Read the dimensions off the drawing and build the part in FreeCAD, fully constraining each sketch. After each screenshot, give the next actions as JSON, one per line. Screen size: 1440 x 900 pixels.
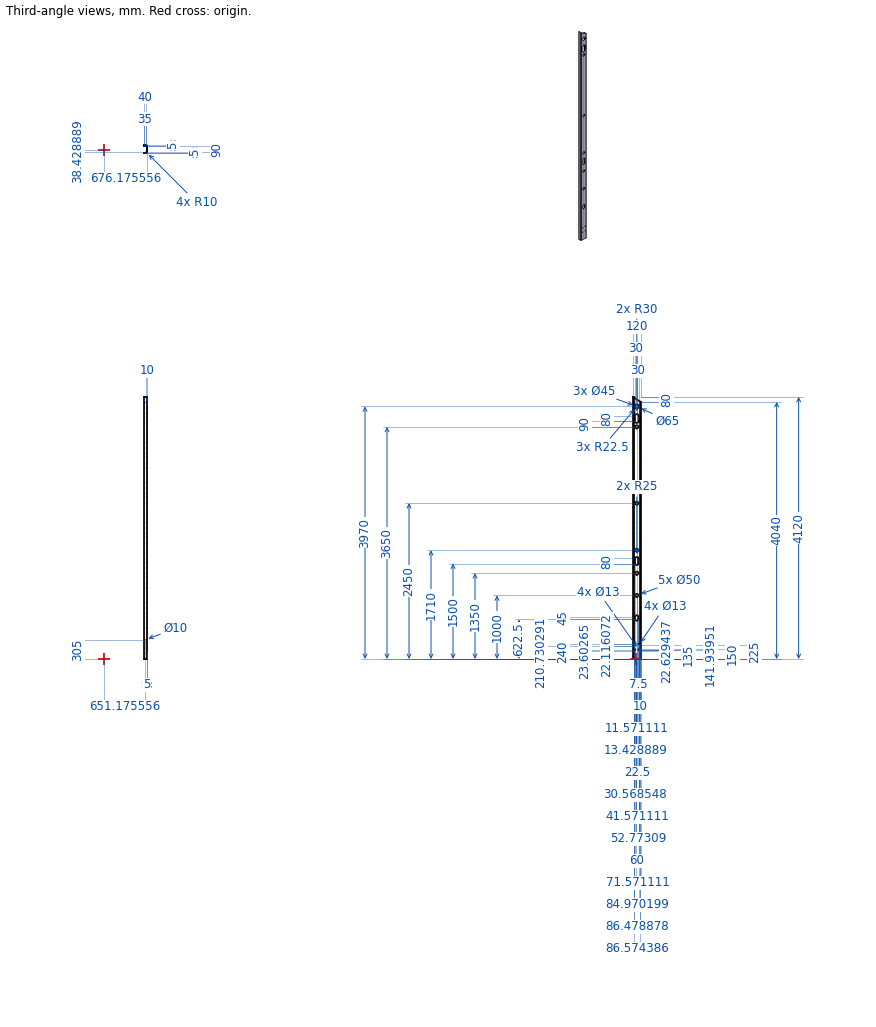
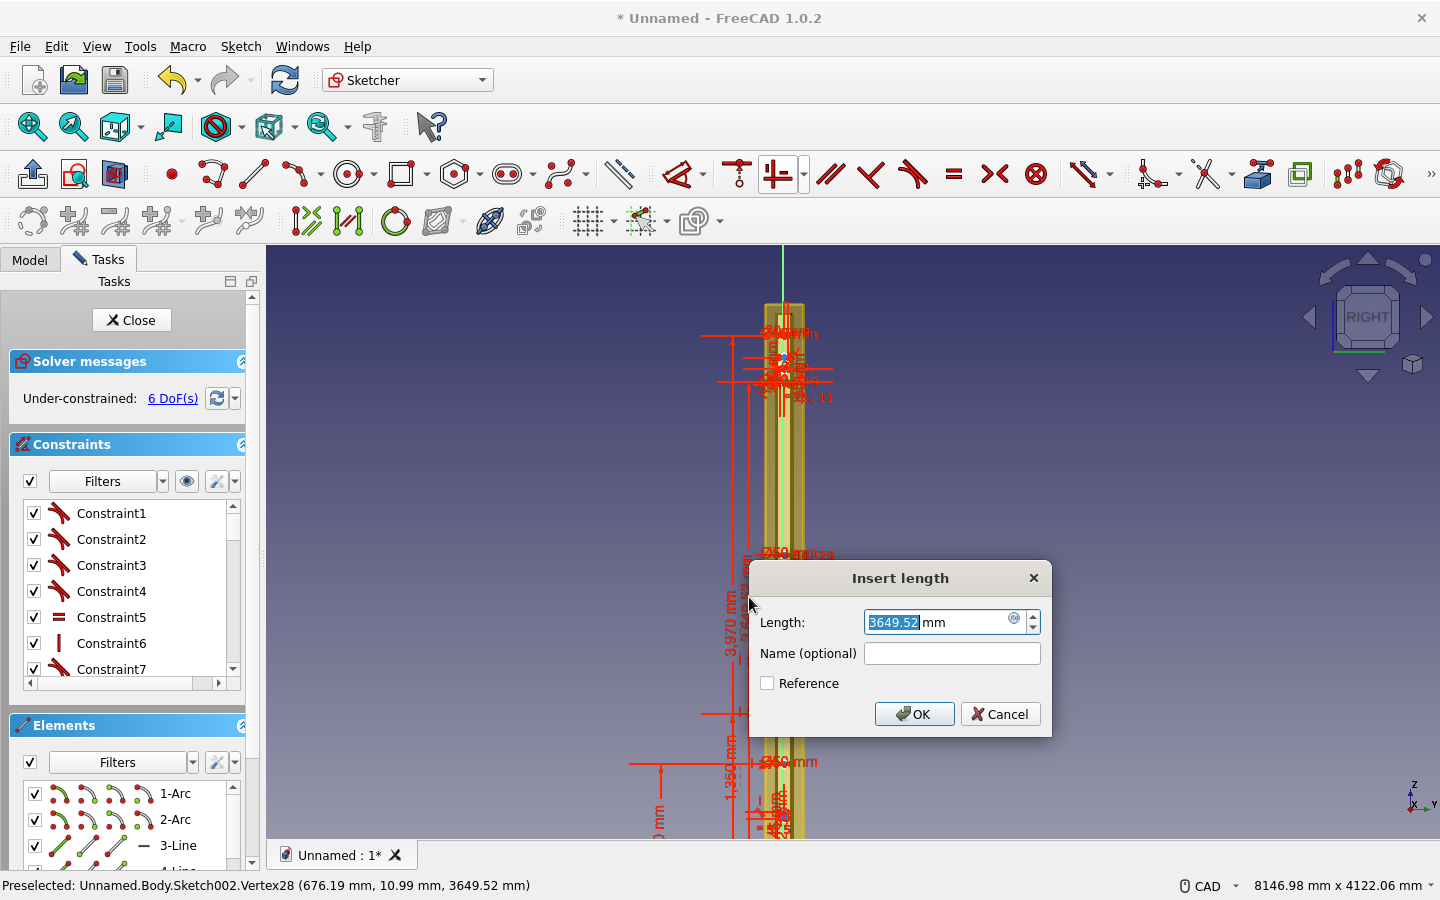
{"action": "type", "text": "3650"}
{"action": "key", "text": "Return"}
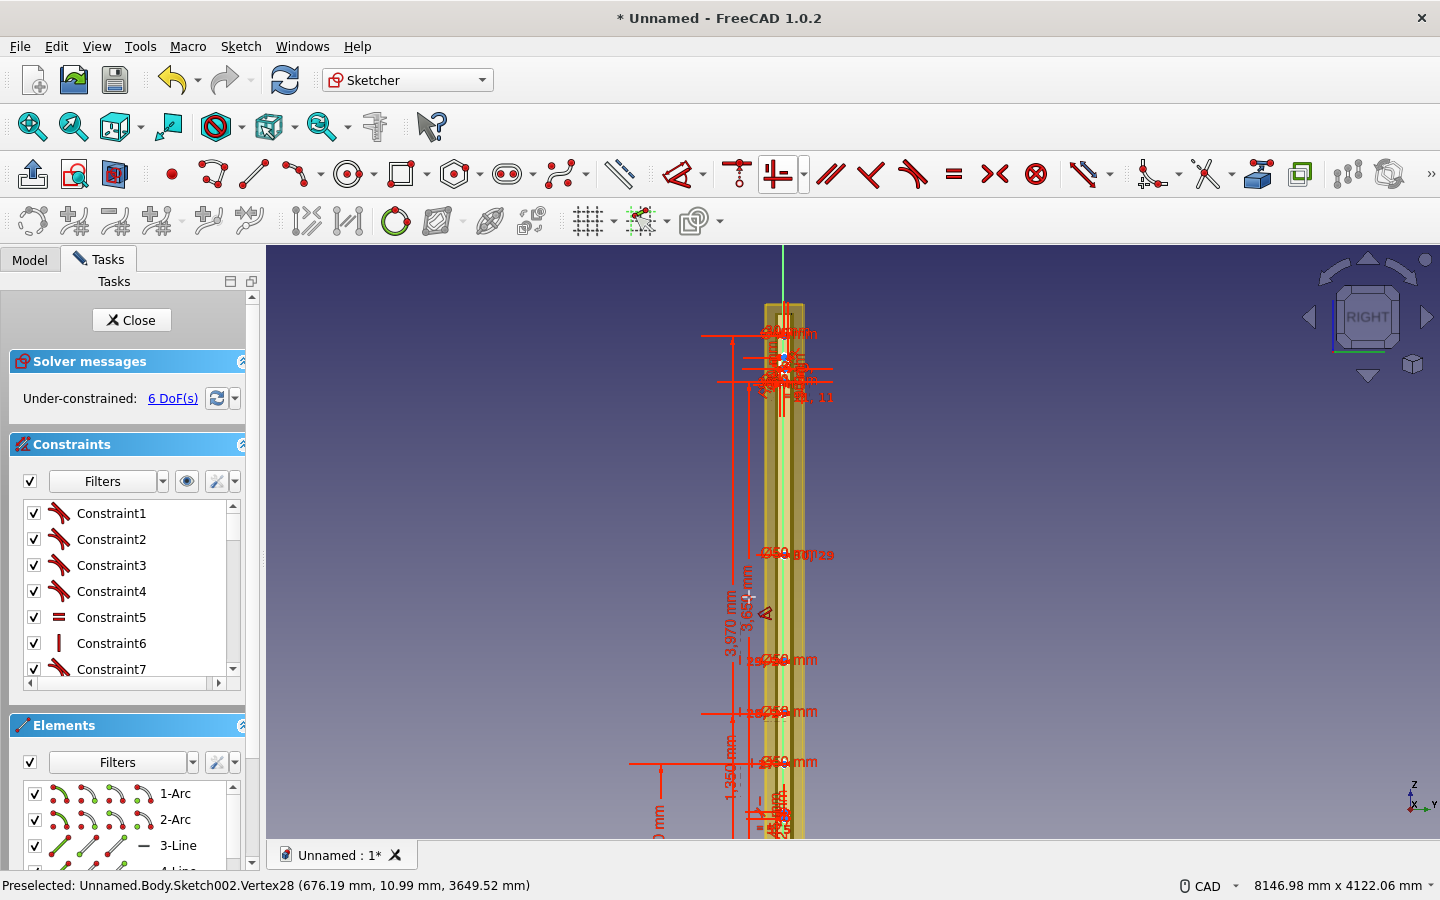
{"action": "left_click", "coordinate": [784, 662]}
{"action": "left_click", "coordinate": [749, 736]}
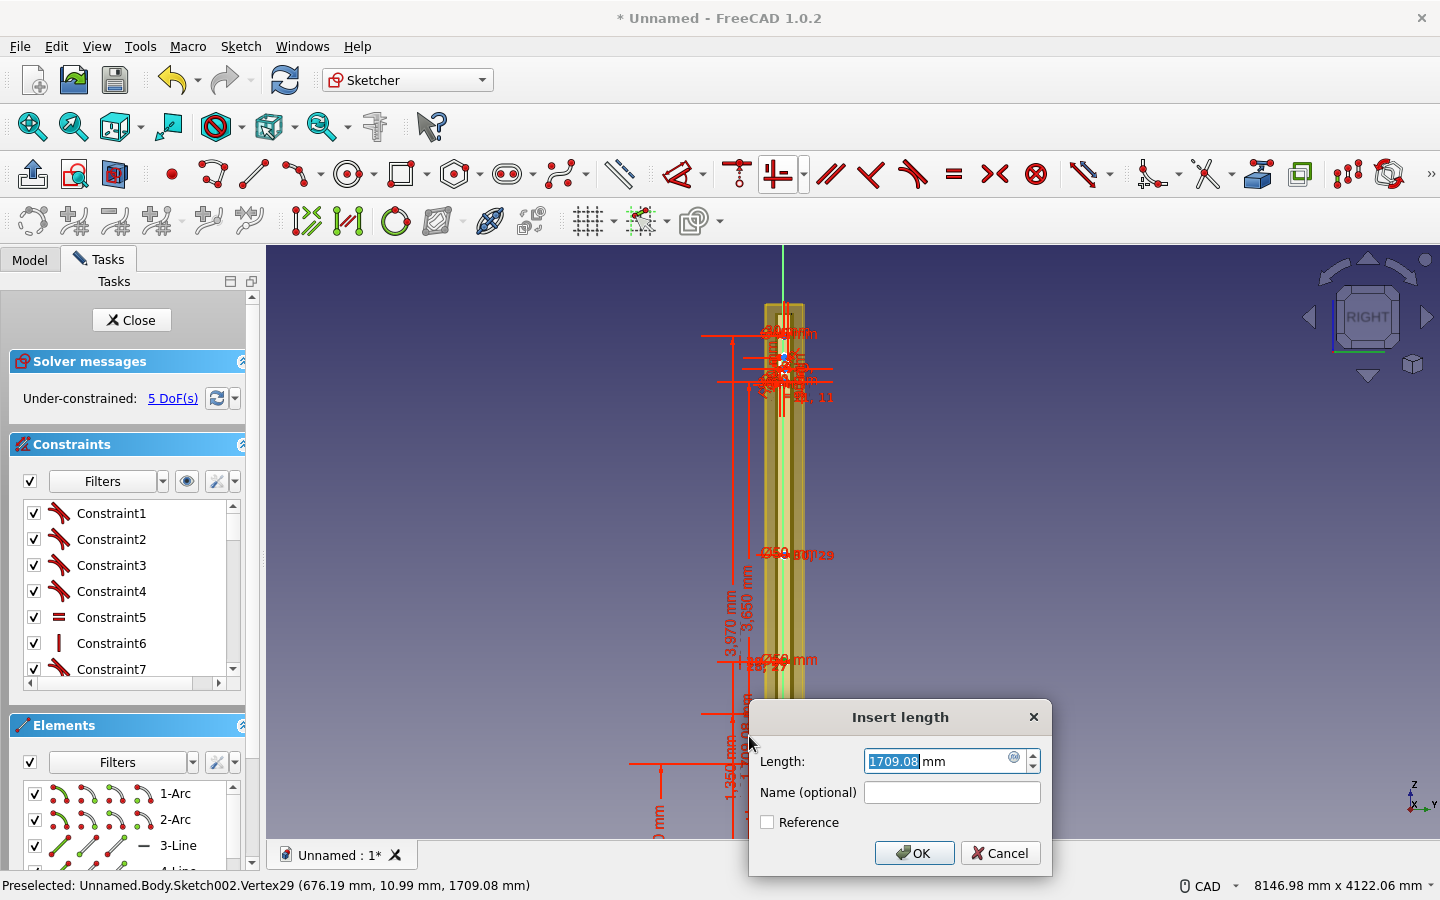
{"action": "type", "text": "1710"}
{"action": "key", "text": "Return"}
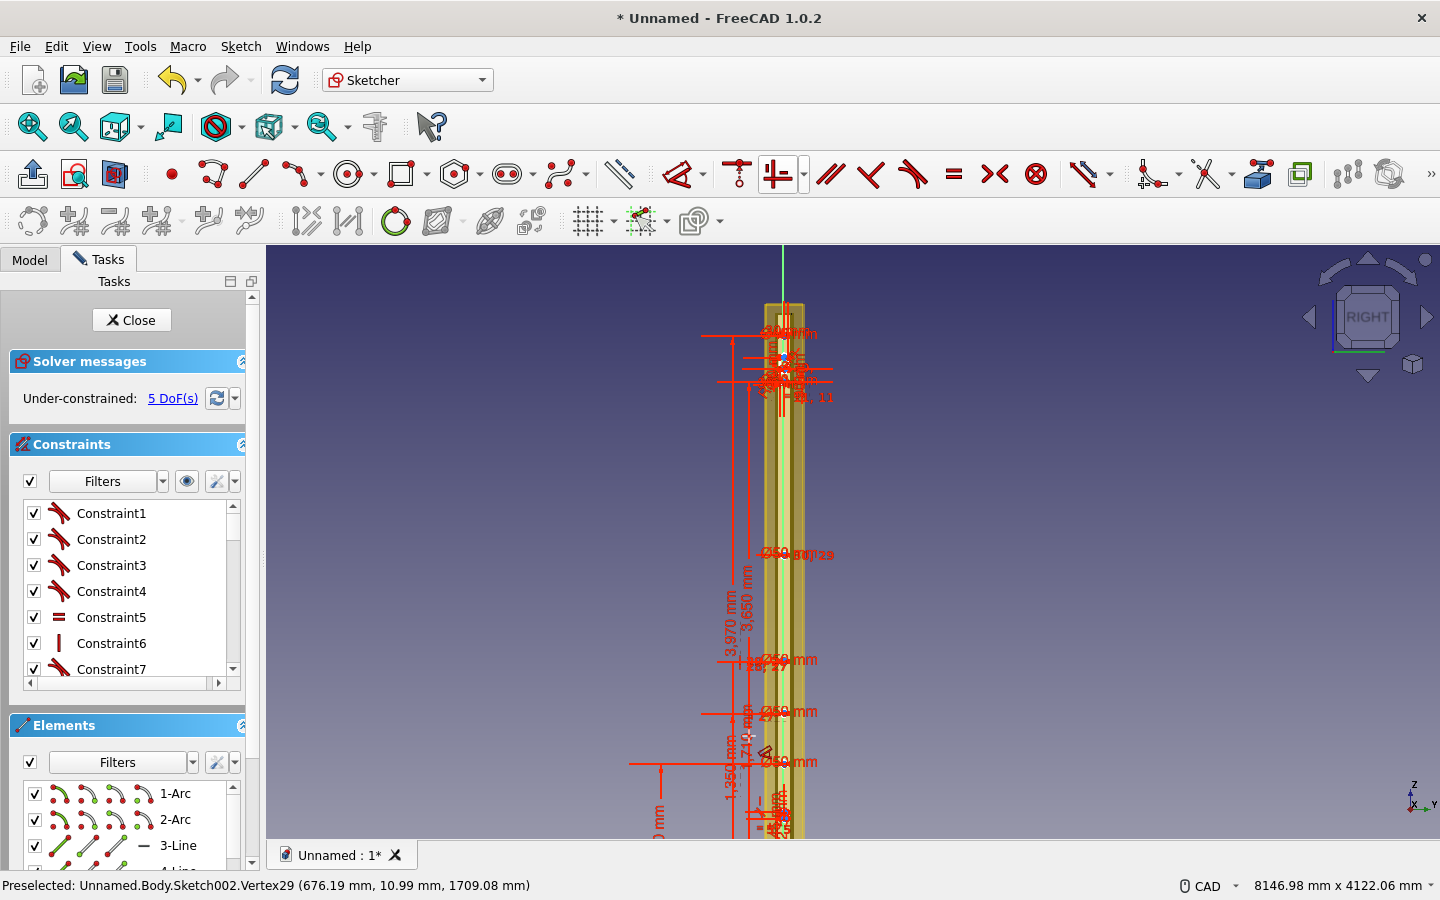
{"action": "left_click", "coordinate": [784, 555]}
{"action": "left_click", "coordinate": [749, 683]}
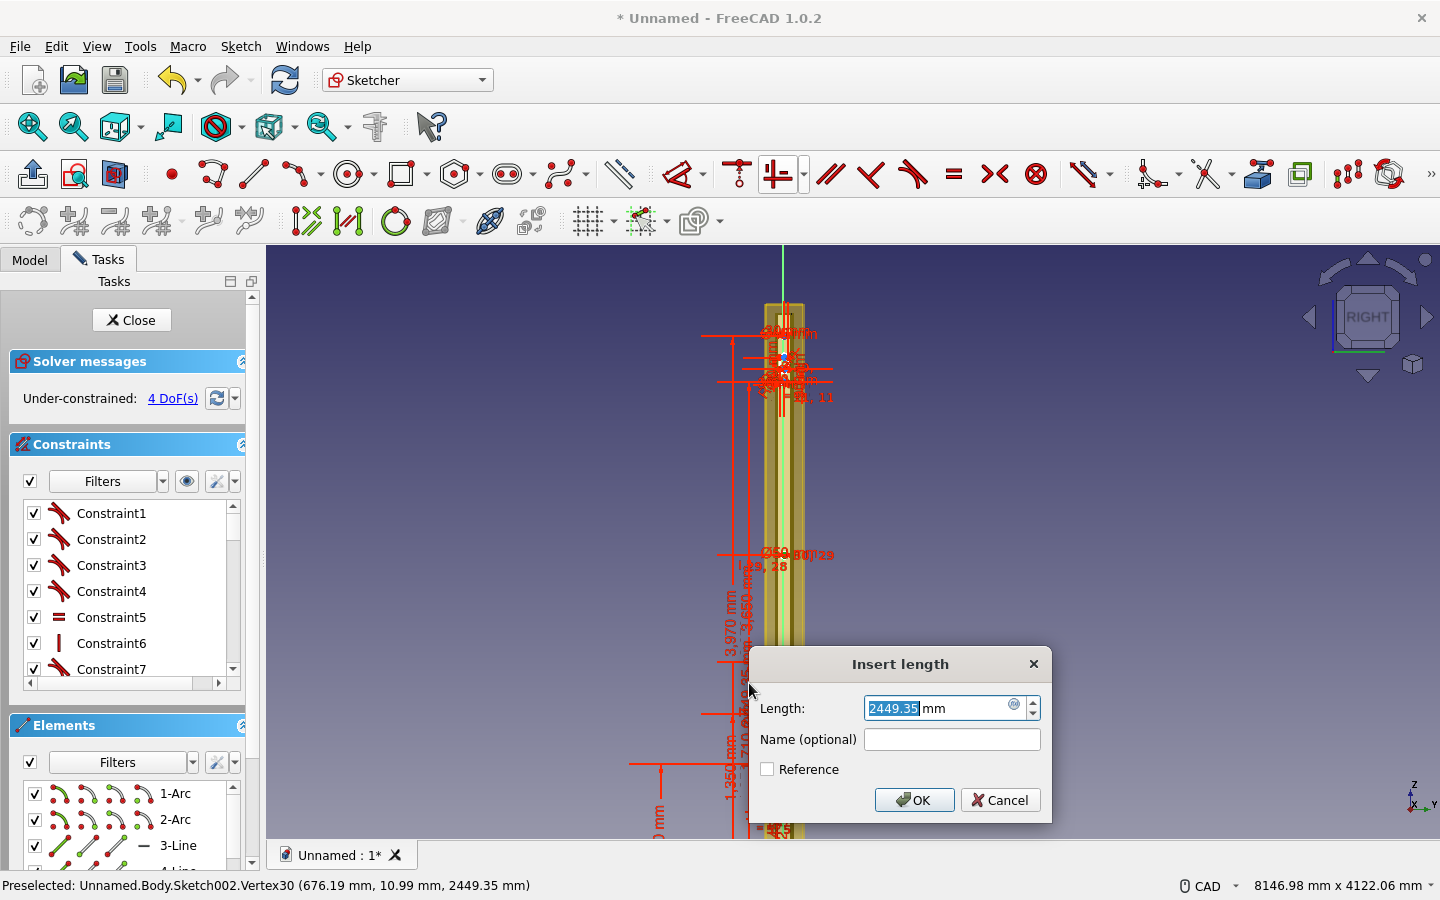
{"action": "type", "text": "2450"}
{"action": "key", "text": "Return"}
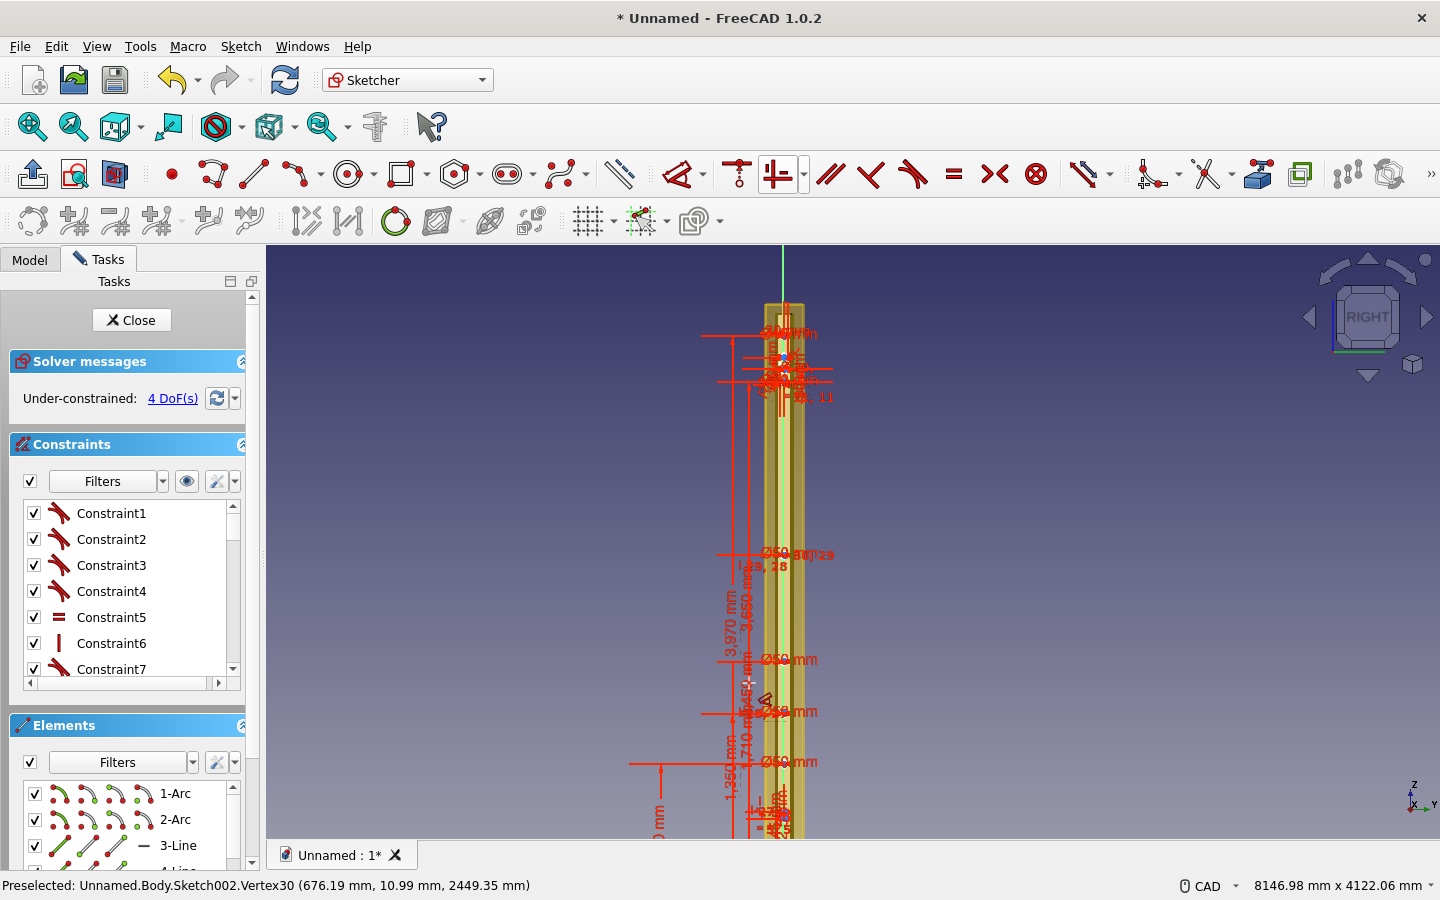
{"action": "scroll", "coordinate": [785, 382], "scroll_direction": "down", "scroll_amount": 2}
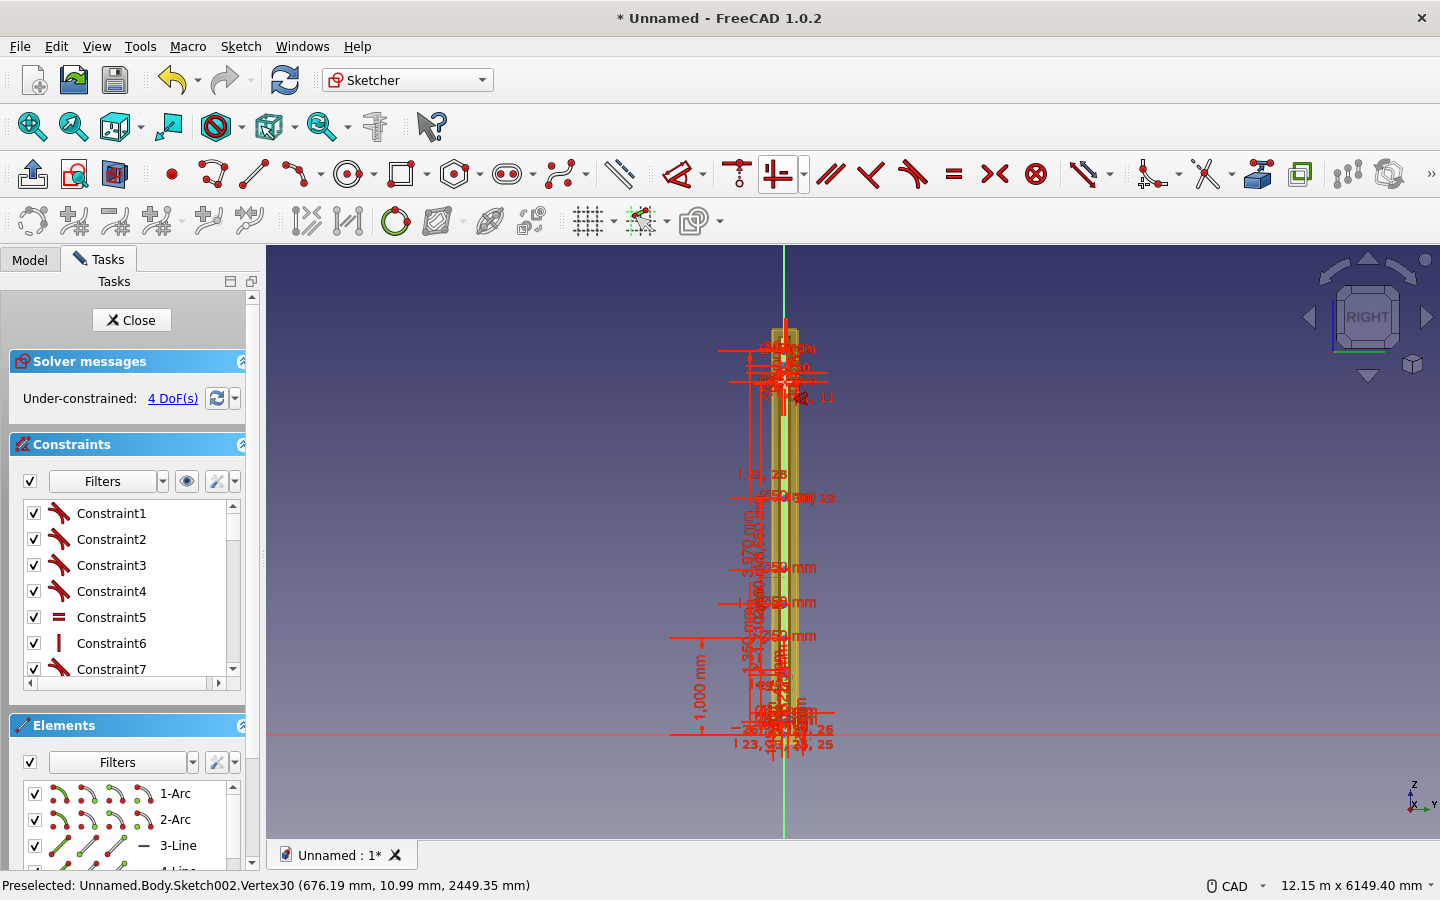
{"action": "scroll", "coordinate": [787, 675], "scroll_direction": "up", "scroll_amount": 21}